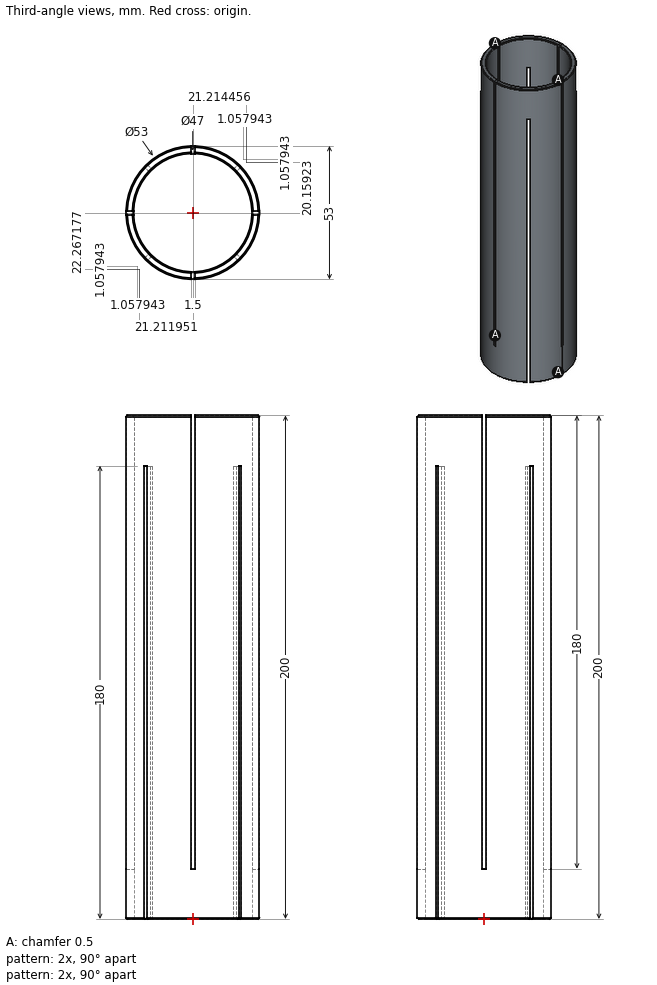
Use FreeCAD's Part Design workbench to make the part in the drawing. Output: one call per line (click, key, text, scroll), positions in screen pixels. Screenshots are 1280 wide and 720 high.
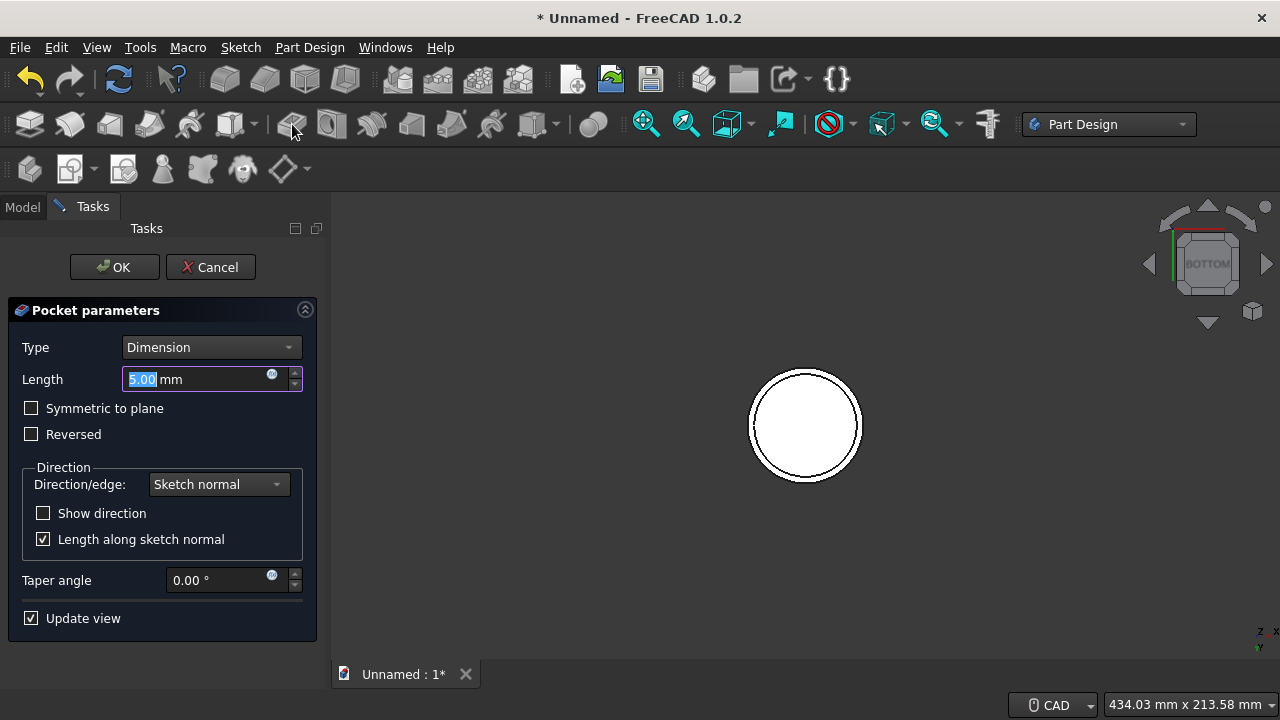
text(200)
key(Tab)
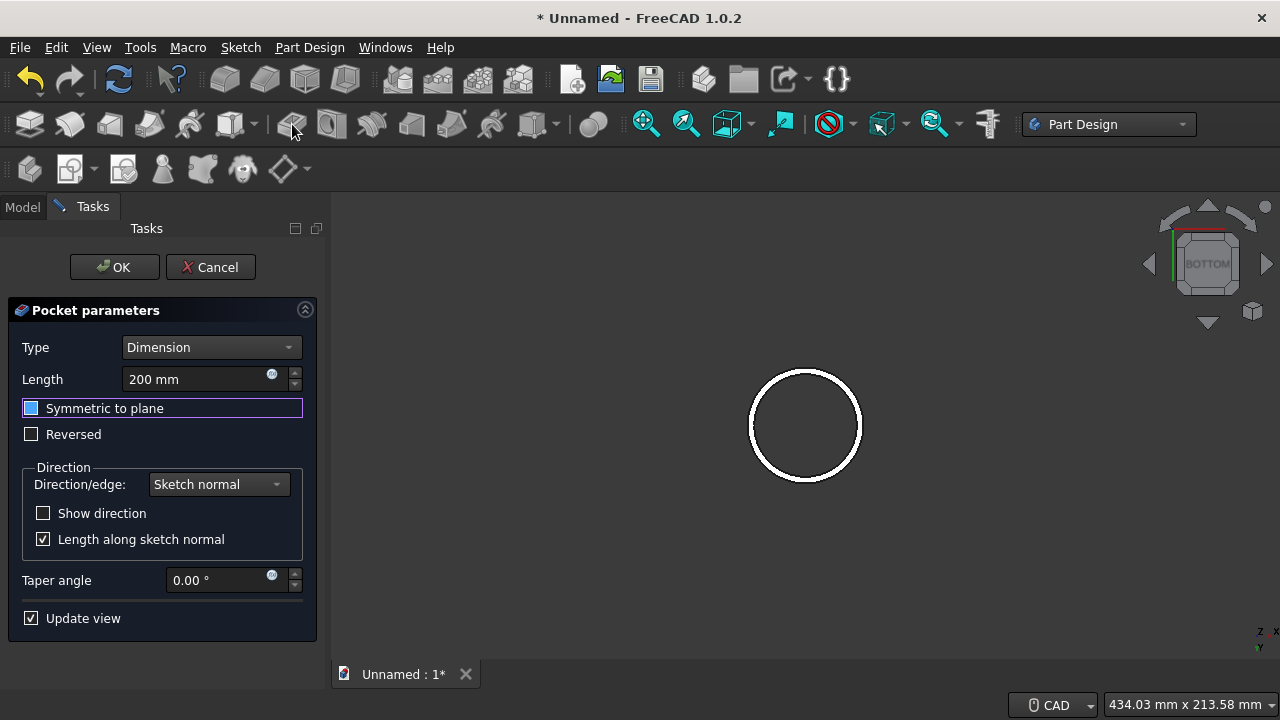
click(115, 267)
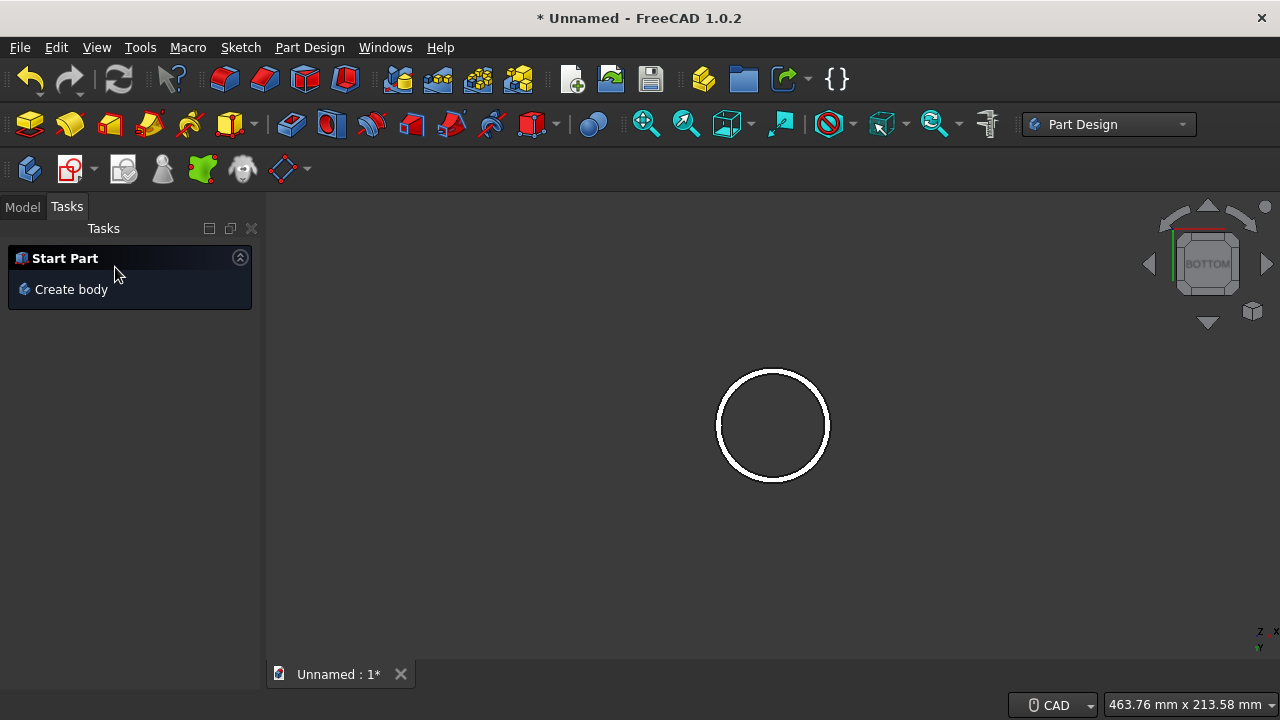
click(648, 124)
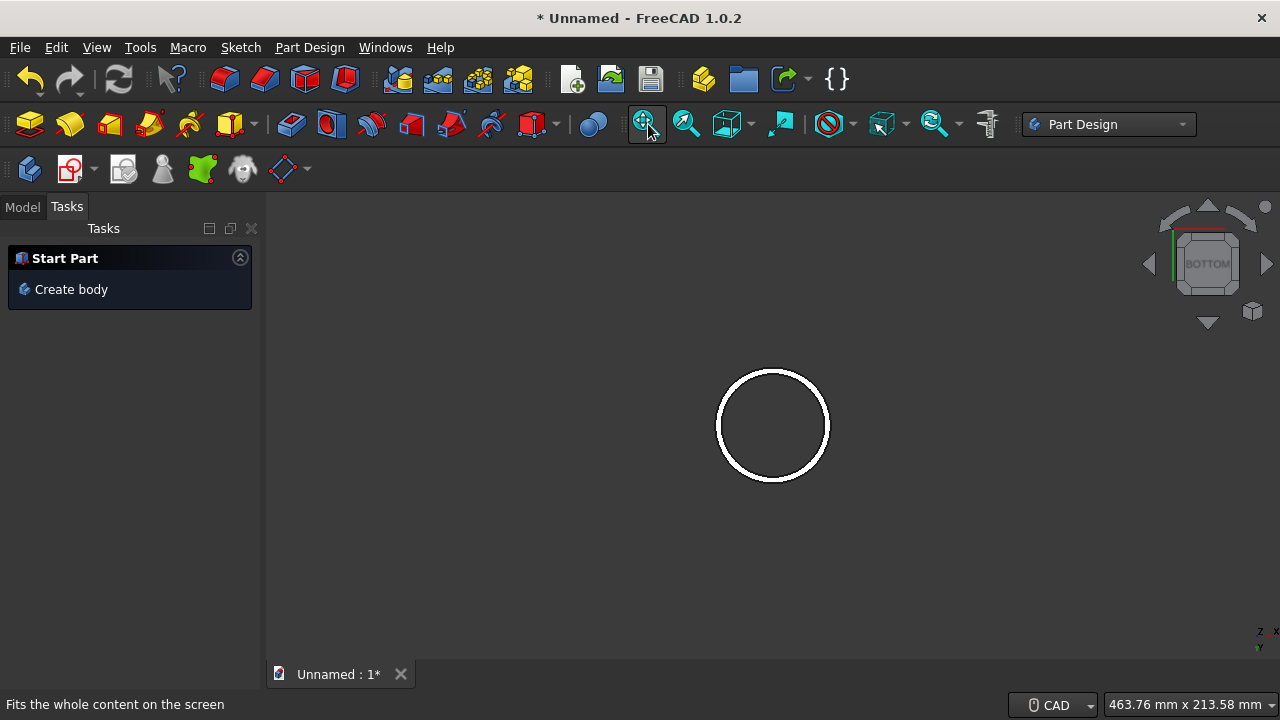
click(715, 424)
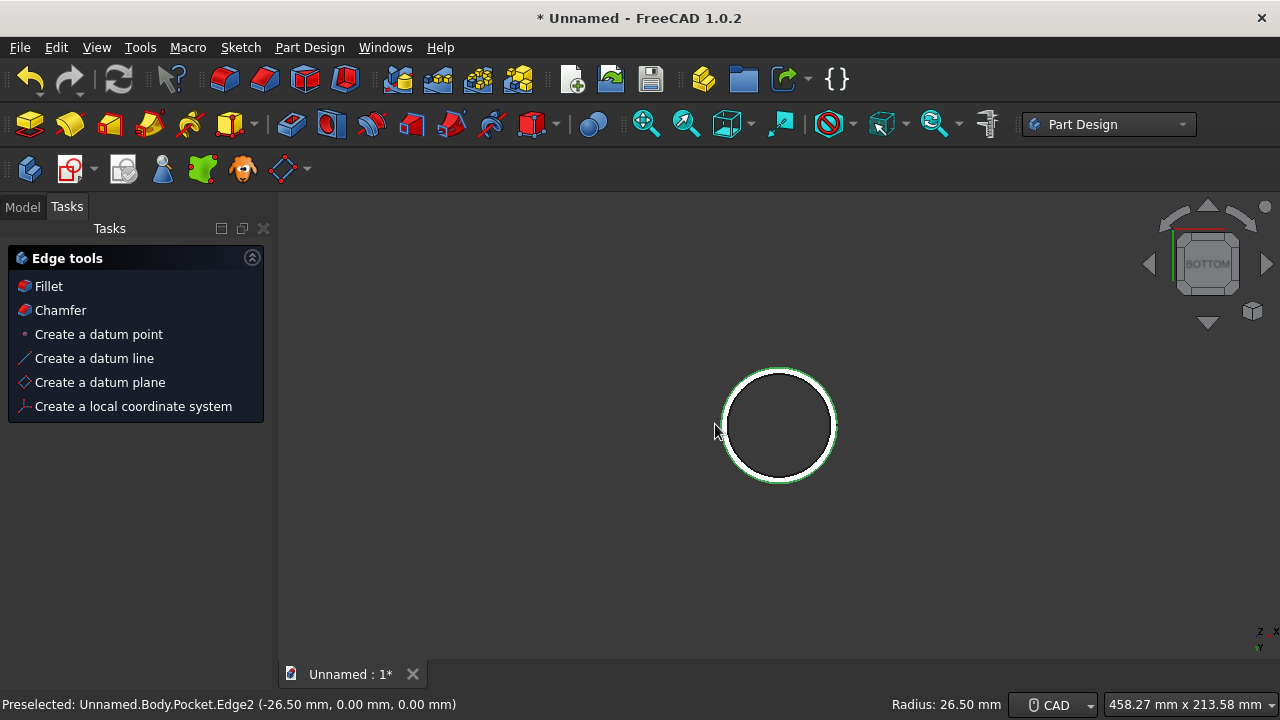
click(737, 394, ctrl)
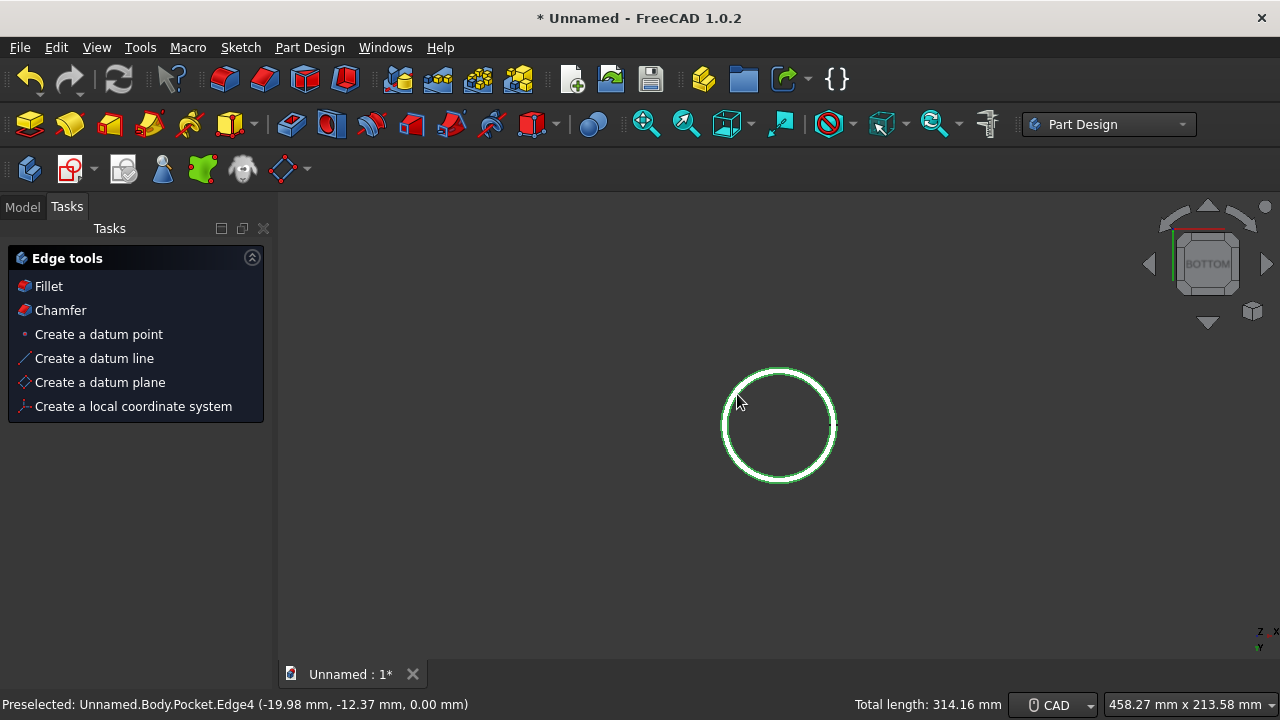
key(0)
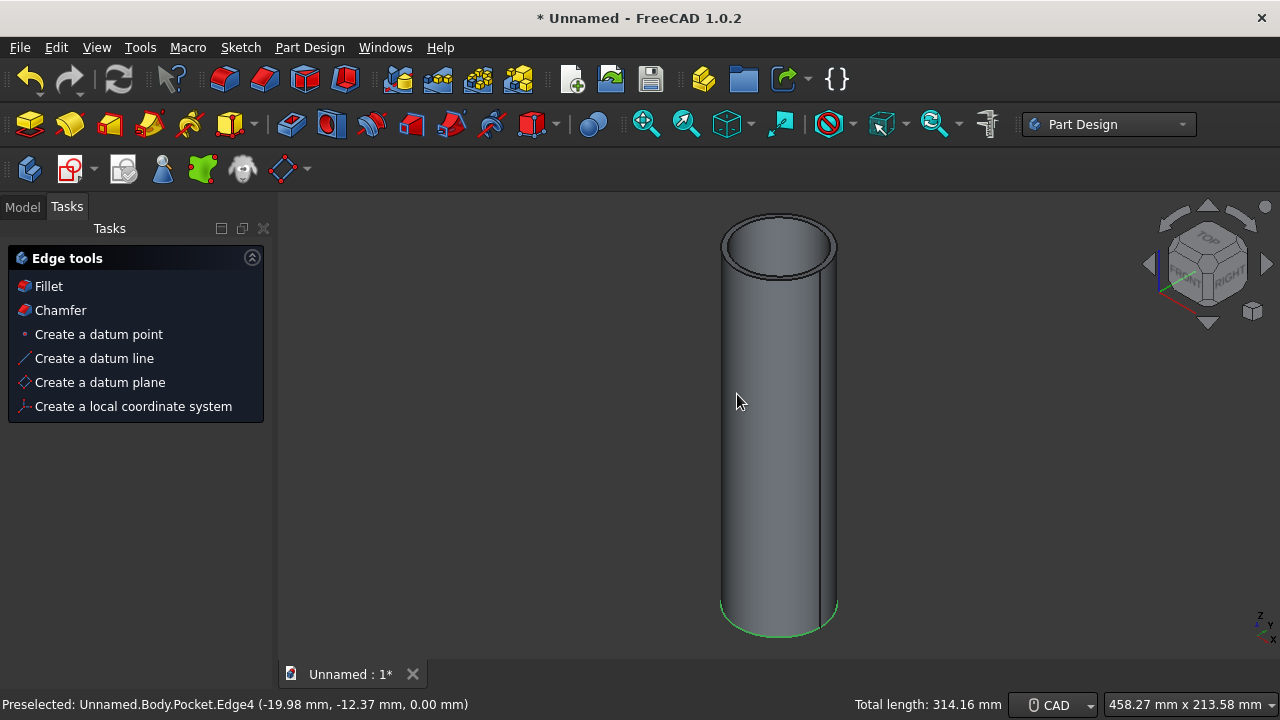
click(727, 261, ctrl)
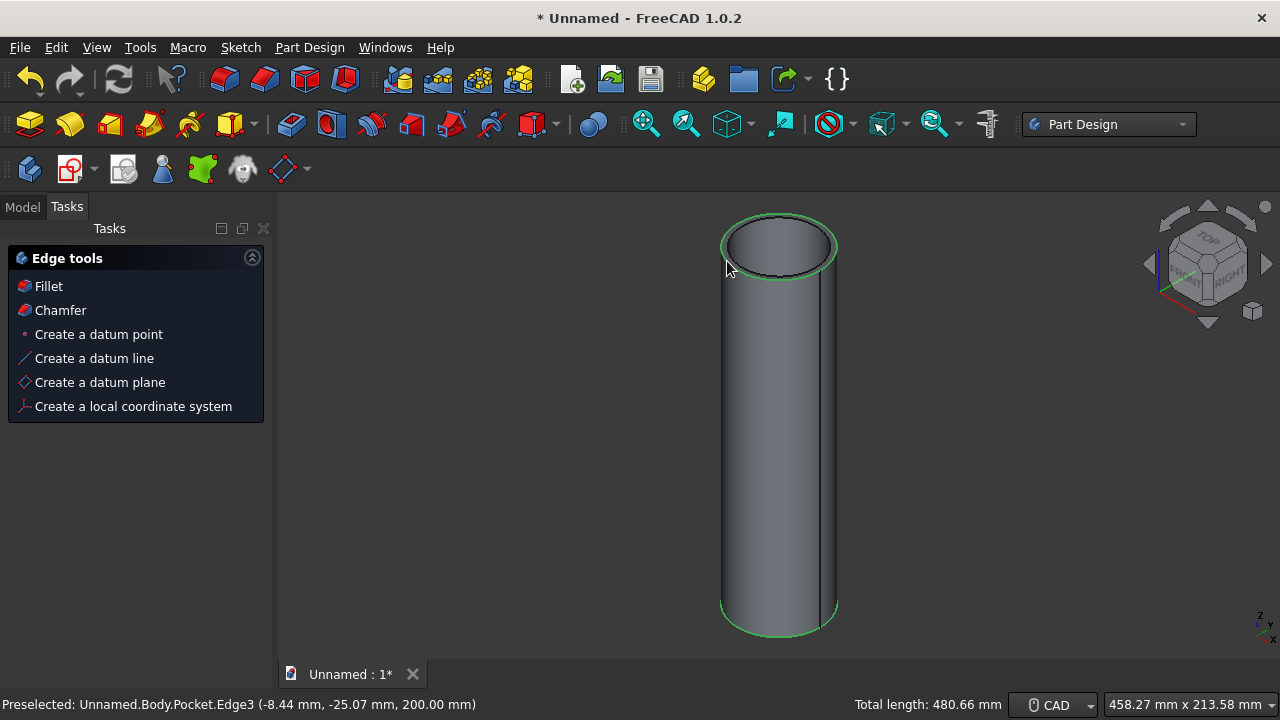
click(743, 225, ctrl)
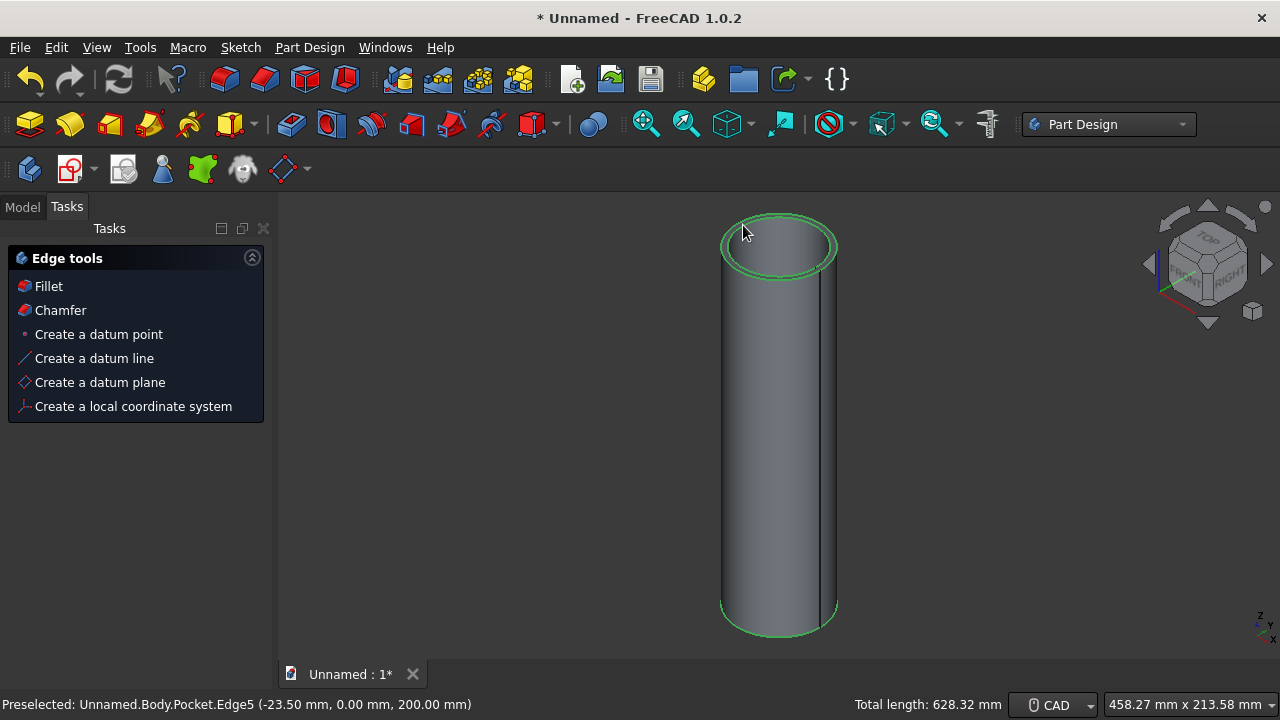
click(266, 80)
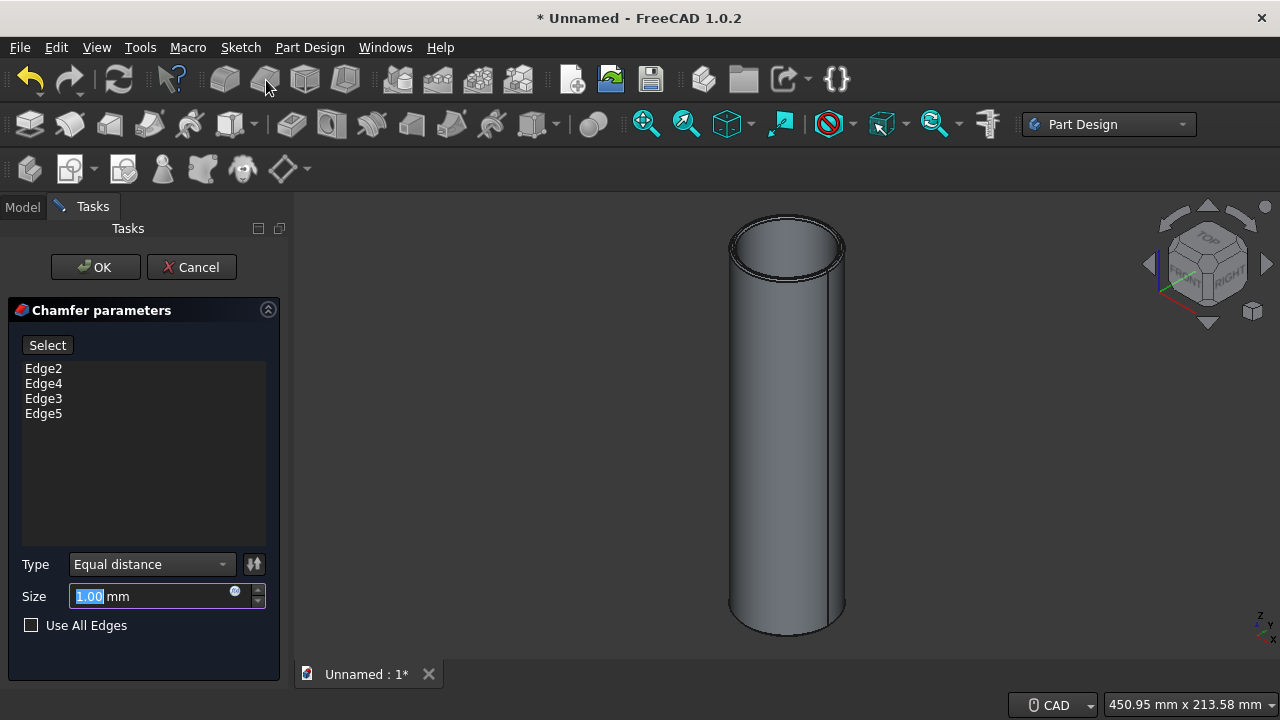
text(0.5)
key(Tab)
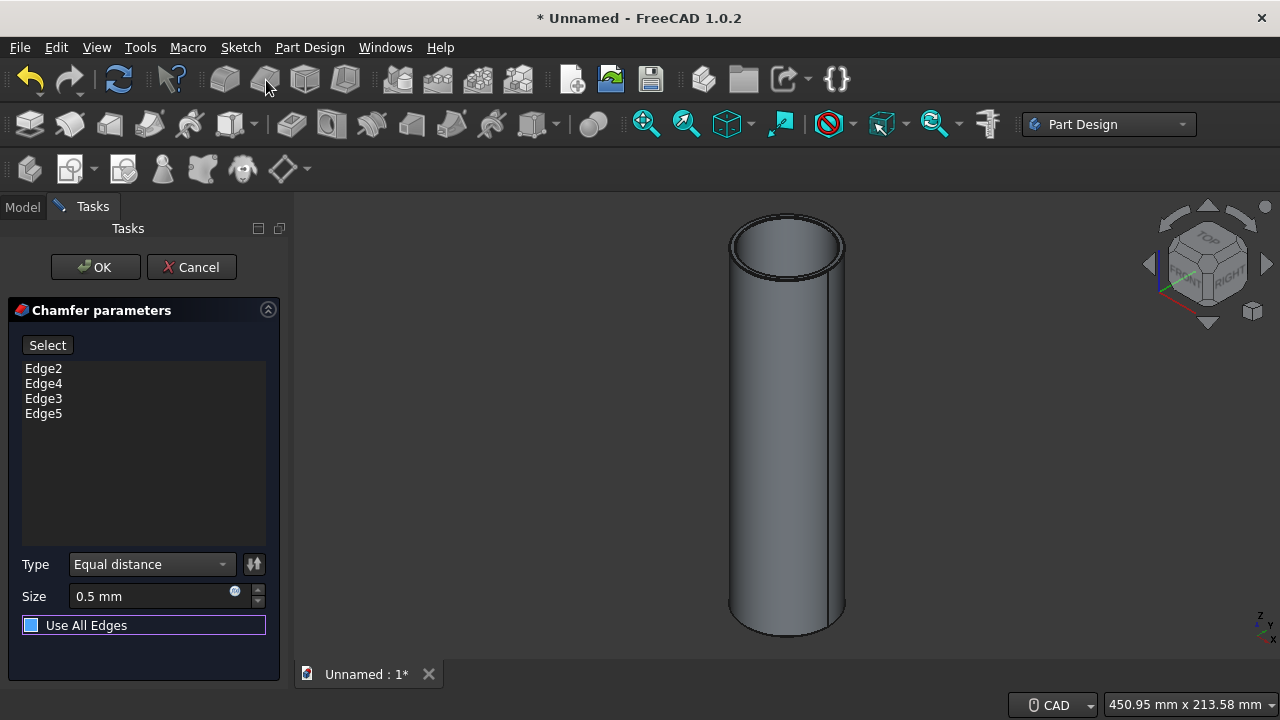
click(96, 267)